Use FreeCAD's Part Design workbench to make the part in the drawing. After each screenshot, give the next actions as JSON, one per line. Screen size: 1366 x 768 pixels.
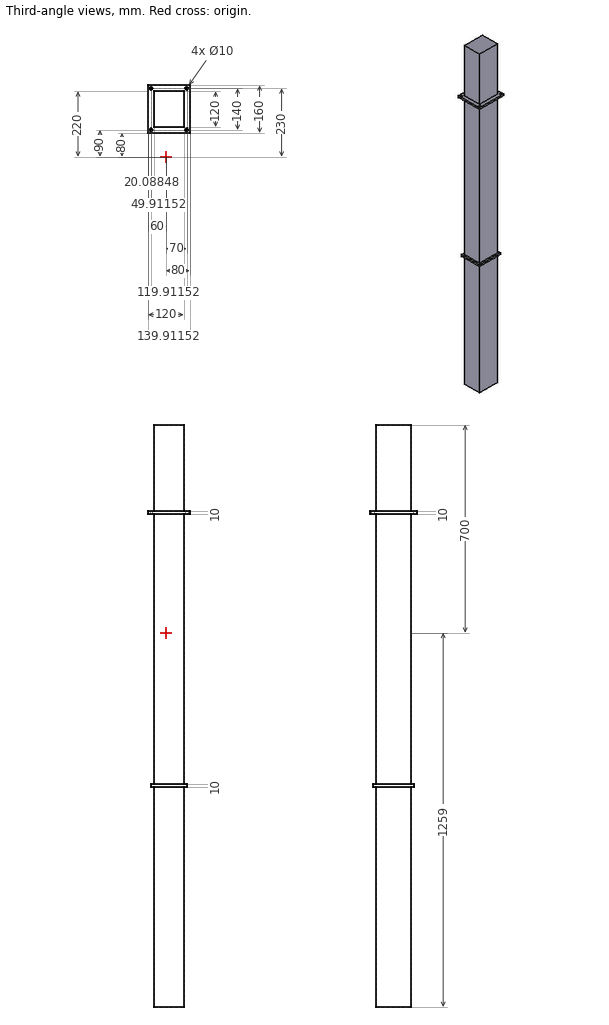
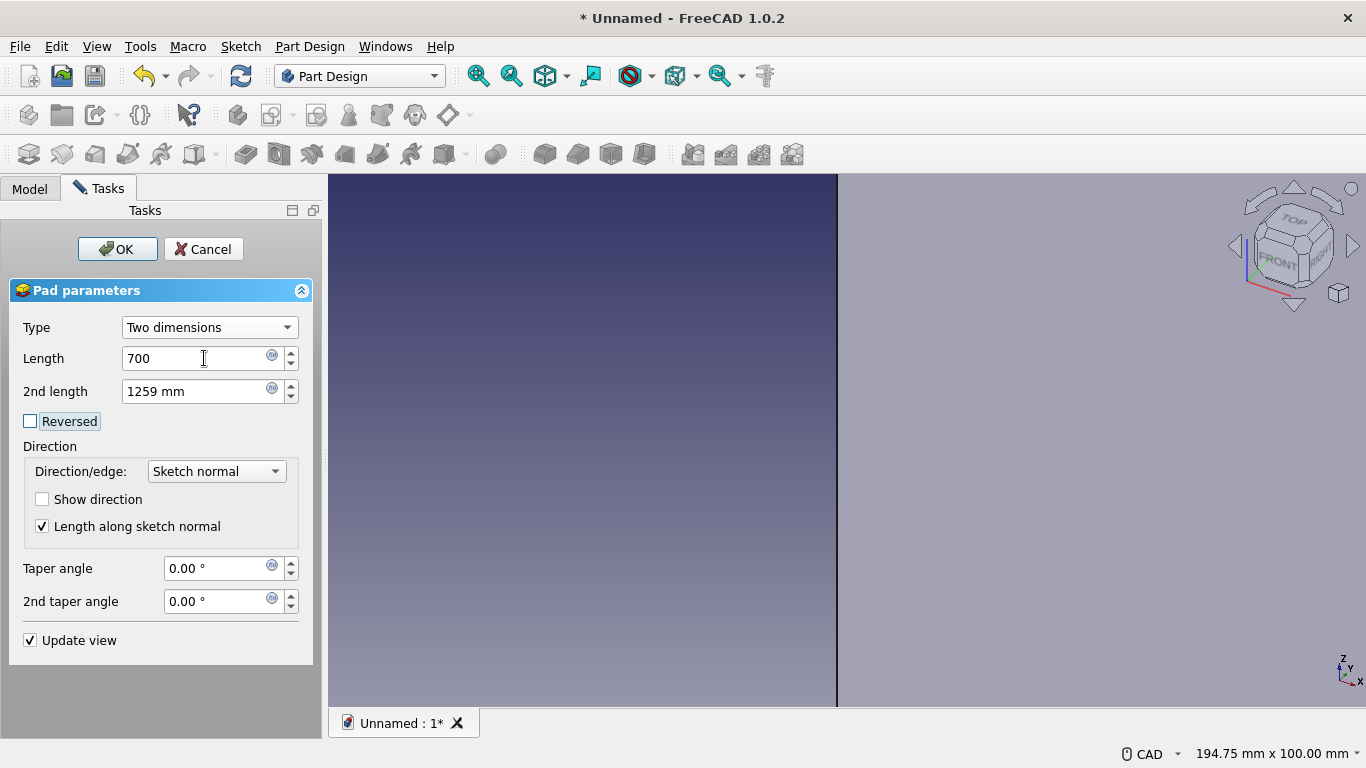
{"action": "left_click", "coordinate": [118, 249]}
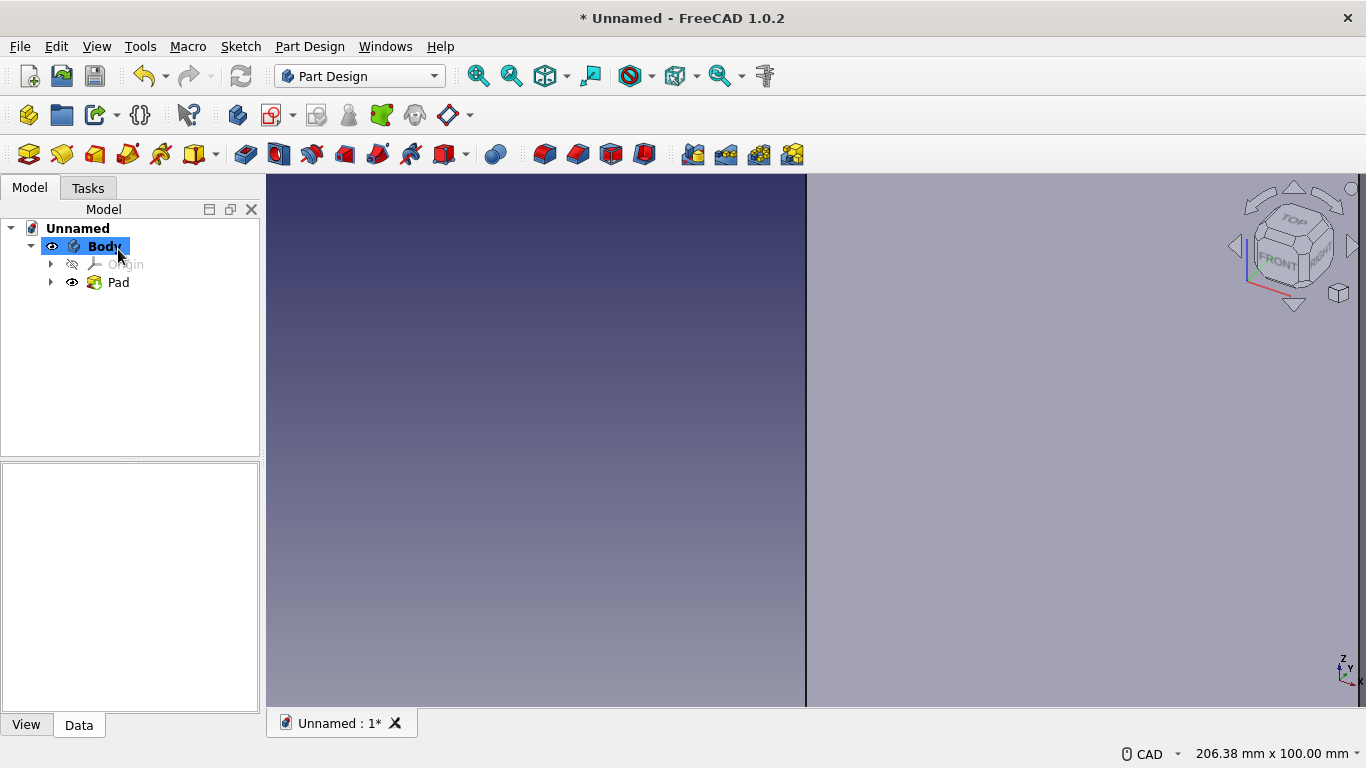
{"action": "key", "text": "v f"}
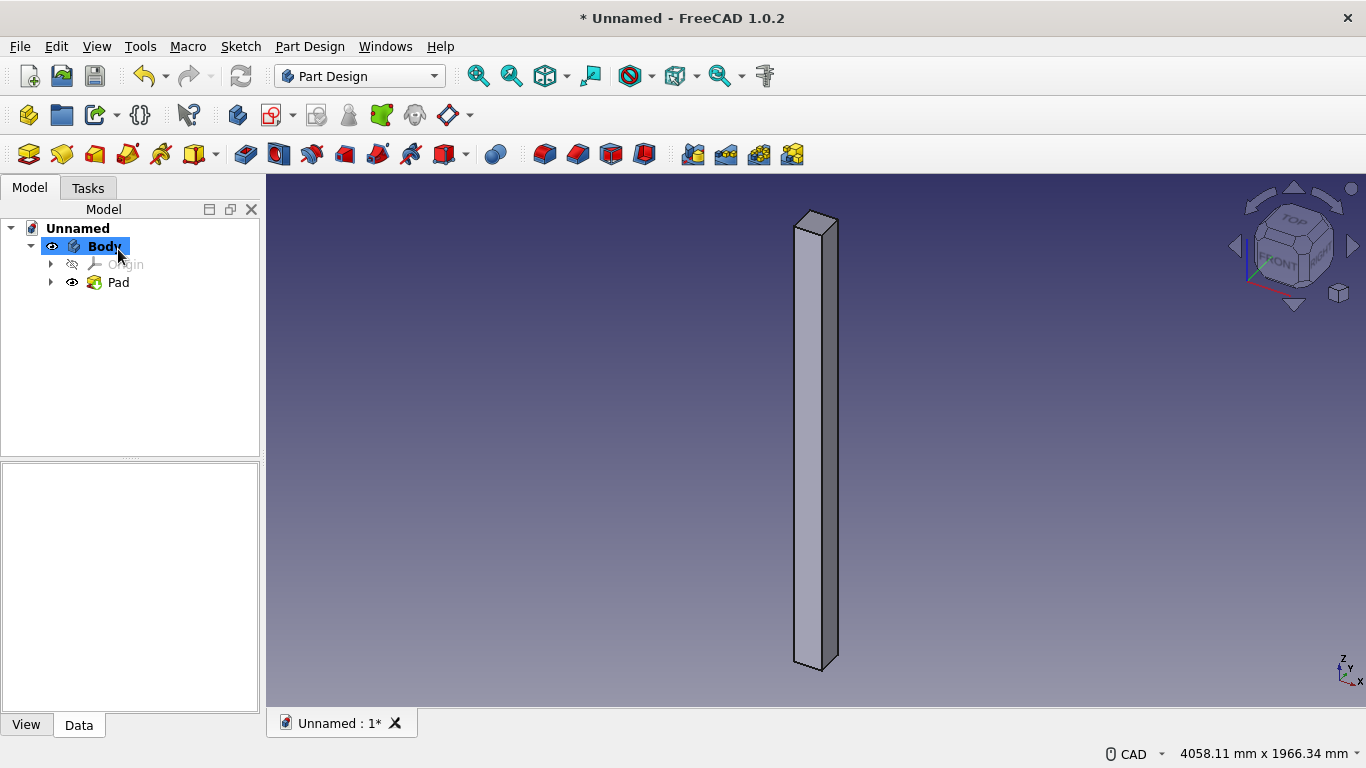
{"action": "left_click", "coordinate": [816, 222]}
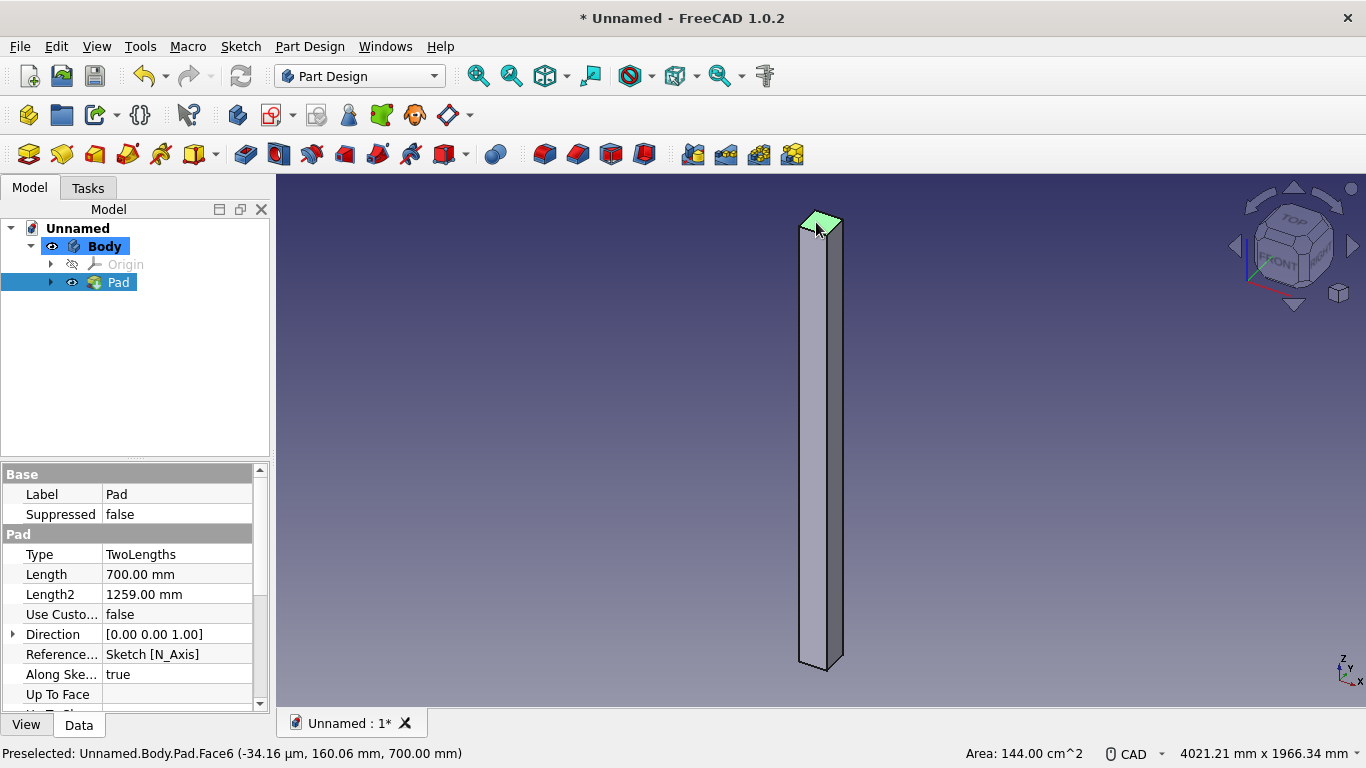
{"action": "left_click", "coordinate": [270, 116]}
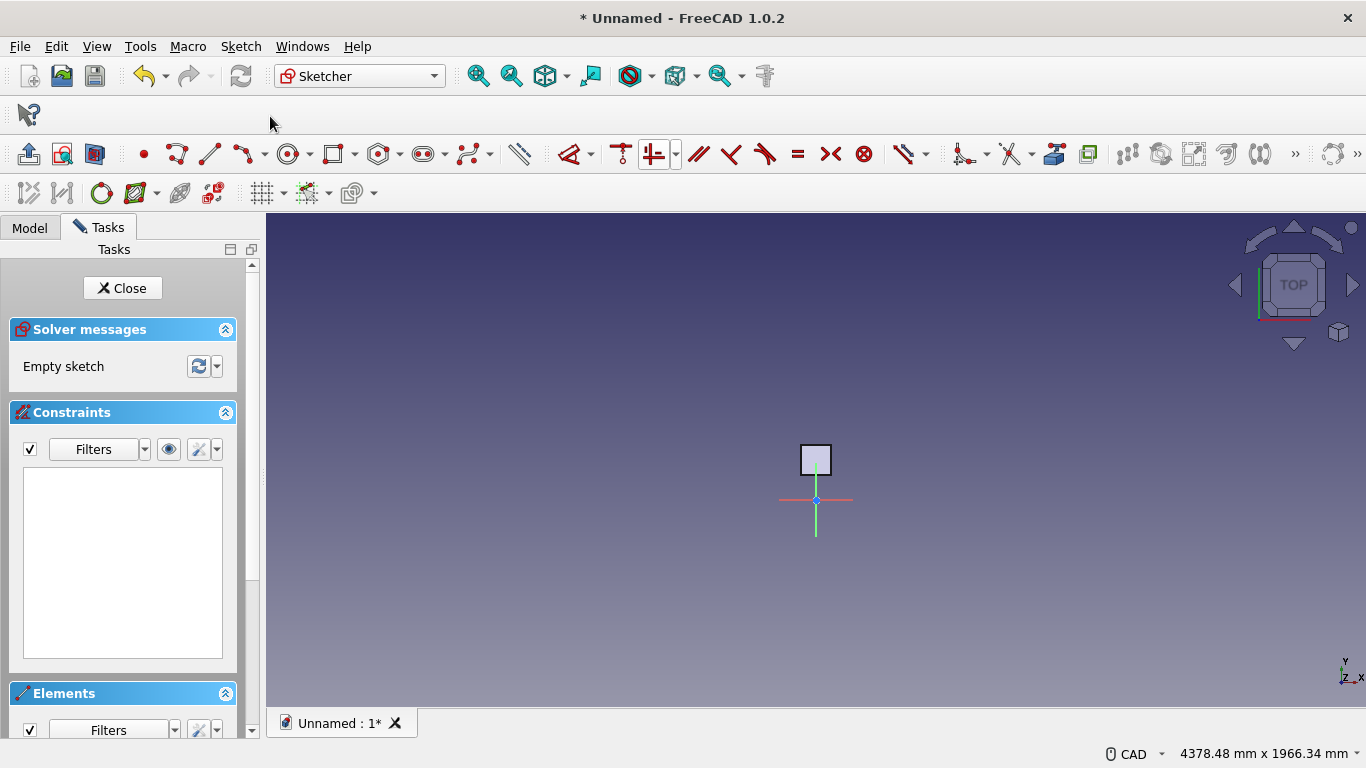
{"action": "scroll", "coordinate": [821, 475], "scroll_direction": "up", "scroll_amount": 9}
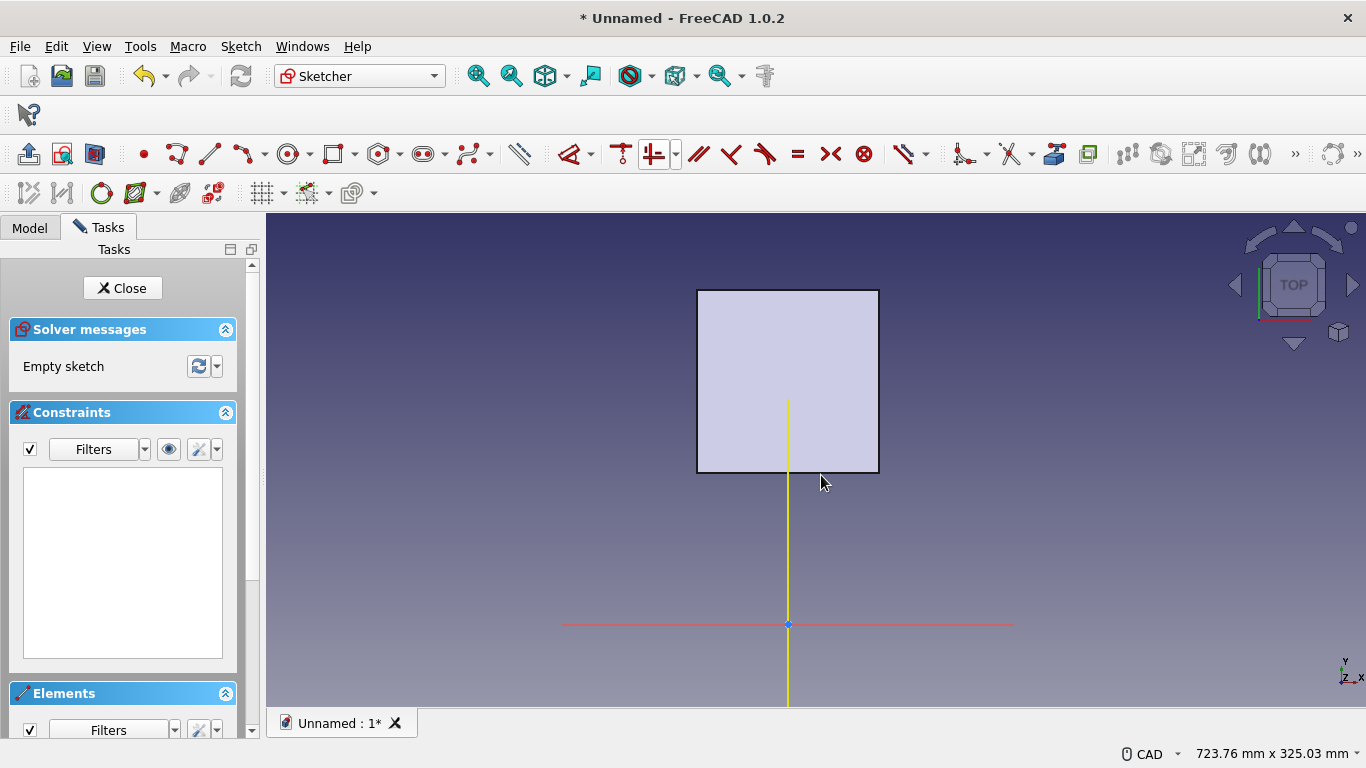
{"action": "key", "text": "g r"}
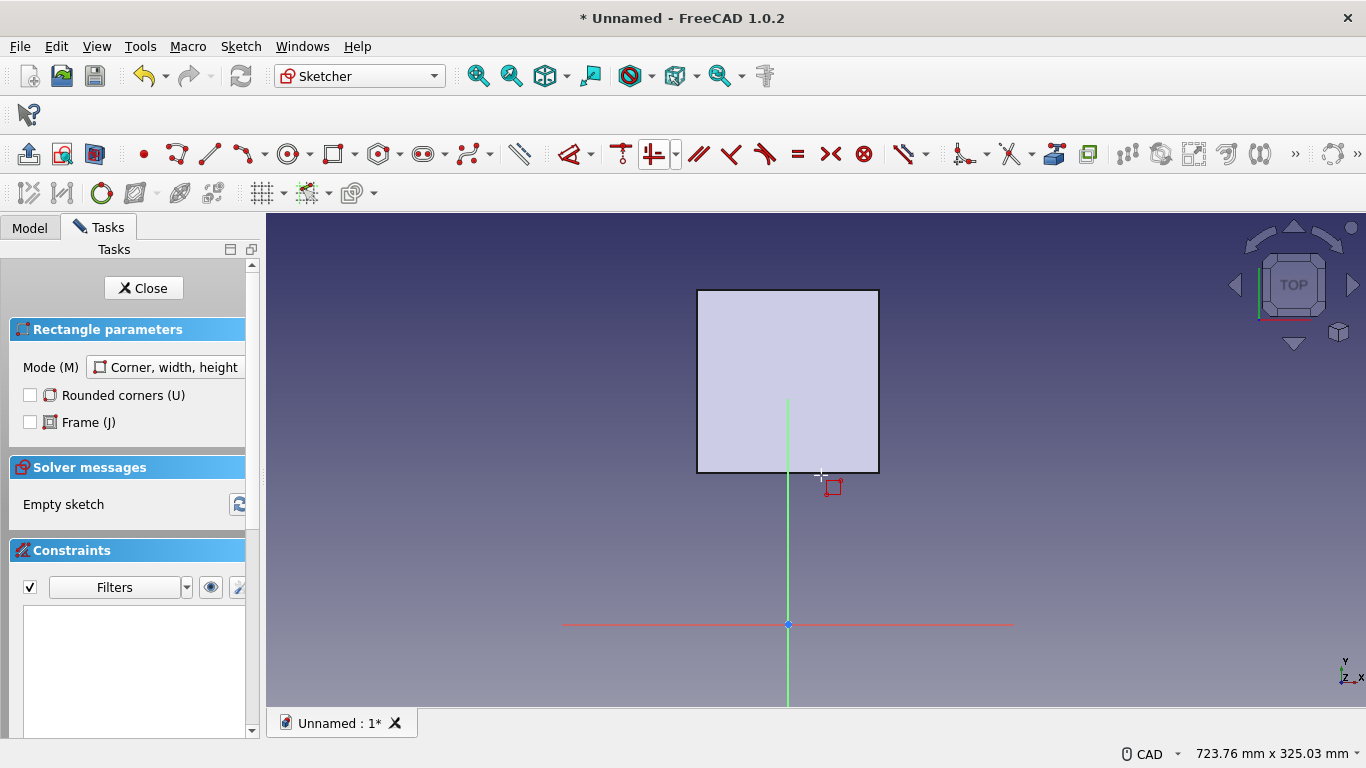
{"action": "left_click", "coordinate": [697, 290]}
{"action": "mouse_move", "coordinate": [728, 473]}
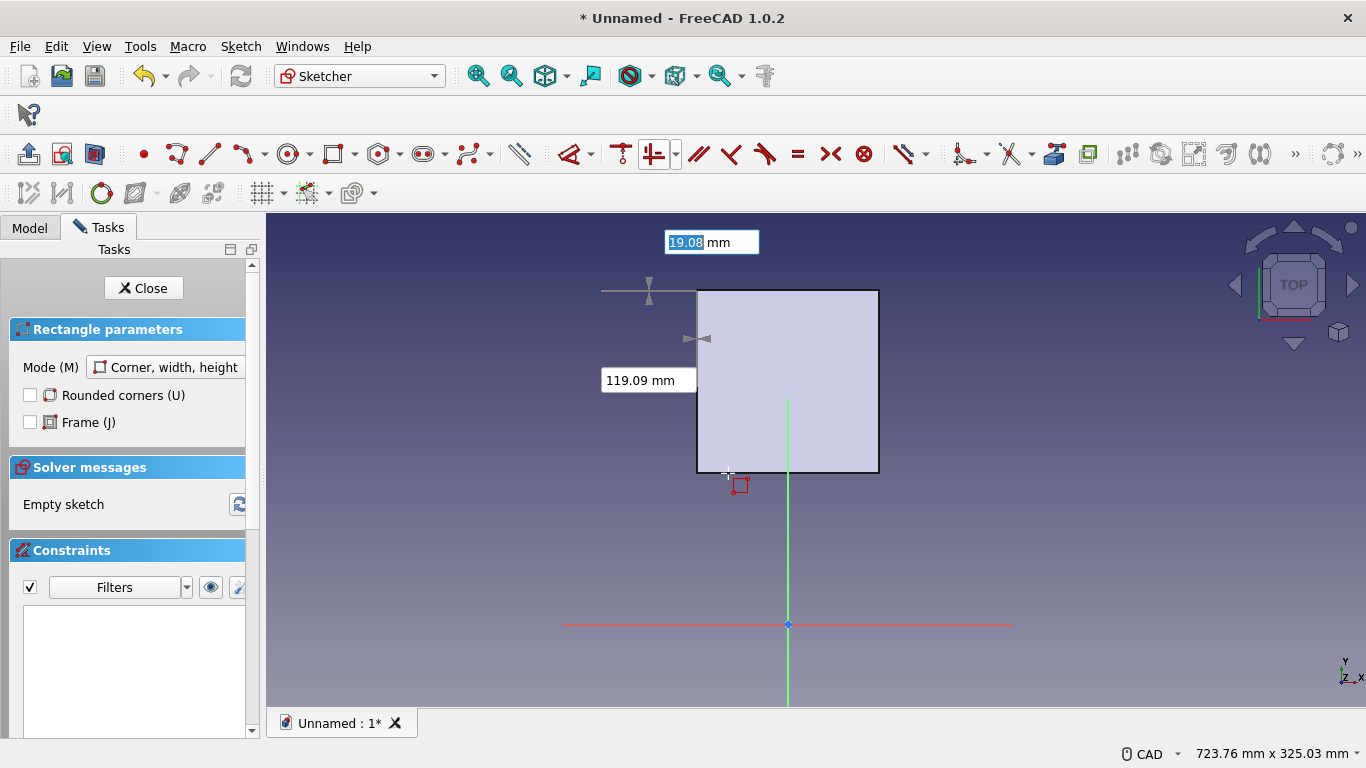
{"action": "type", "text": "20.08848"}
{"action": "key", "text": "Tab"}
{"action": "type", "text": "120"}
{"action": "key", "text": "Return"}
{"action": "key", "text": "Escape"}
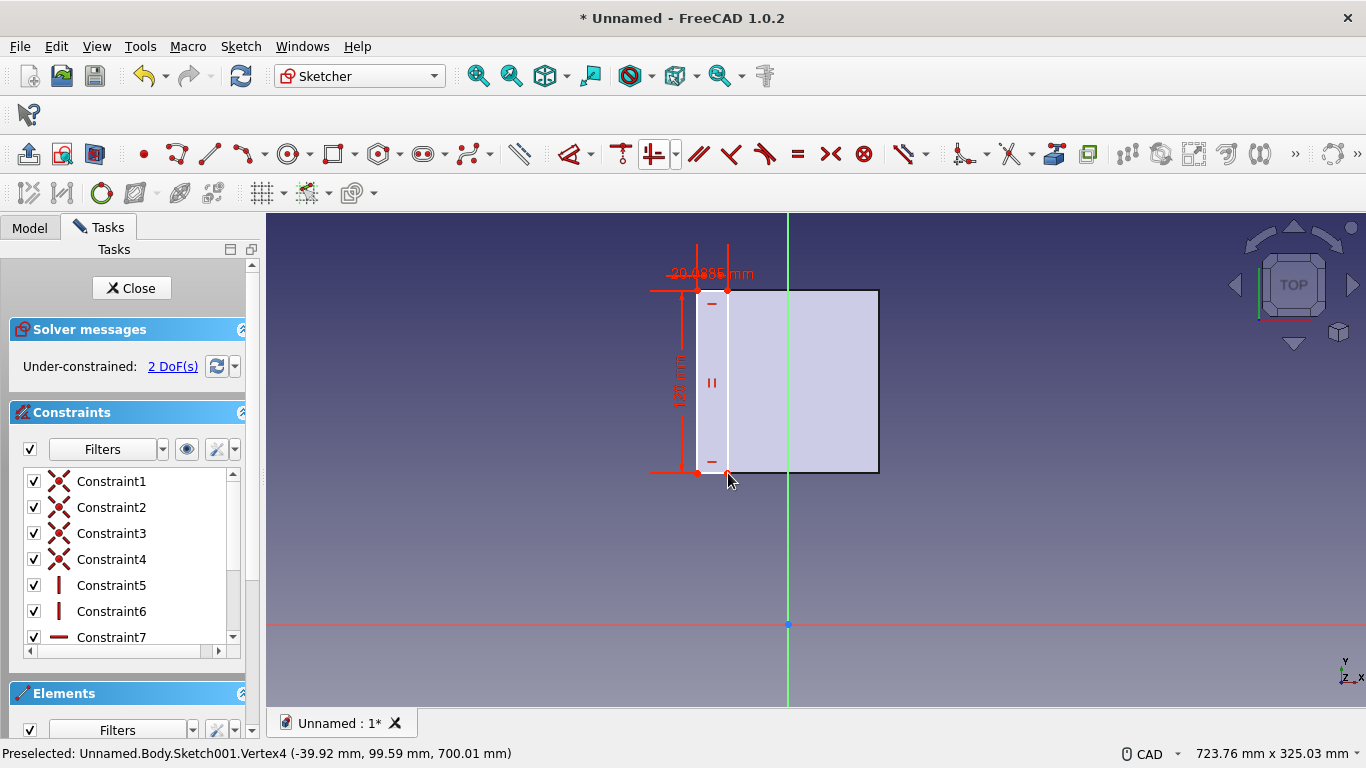
{"action": "left_click", "coordinate": [568, 154]}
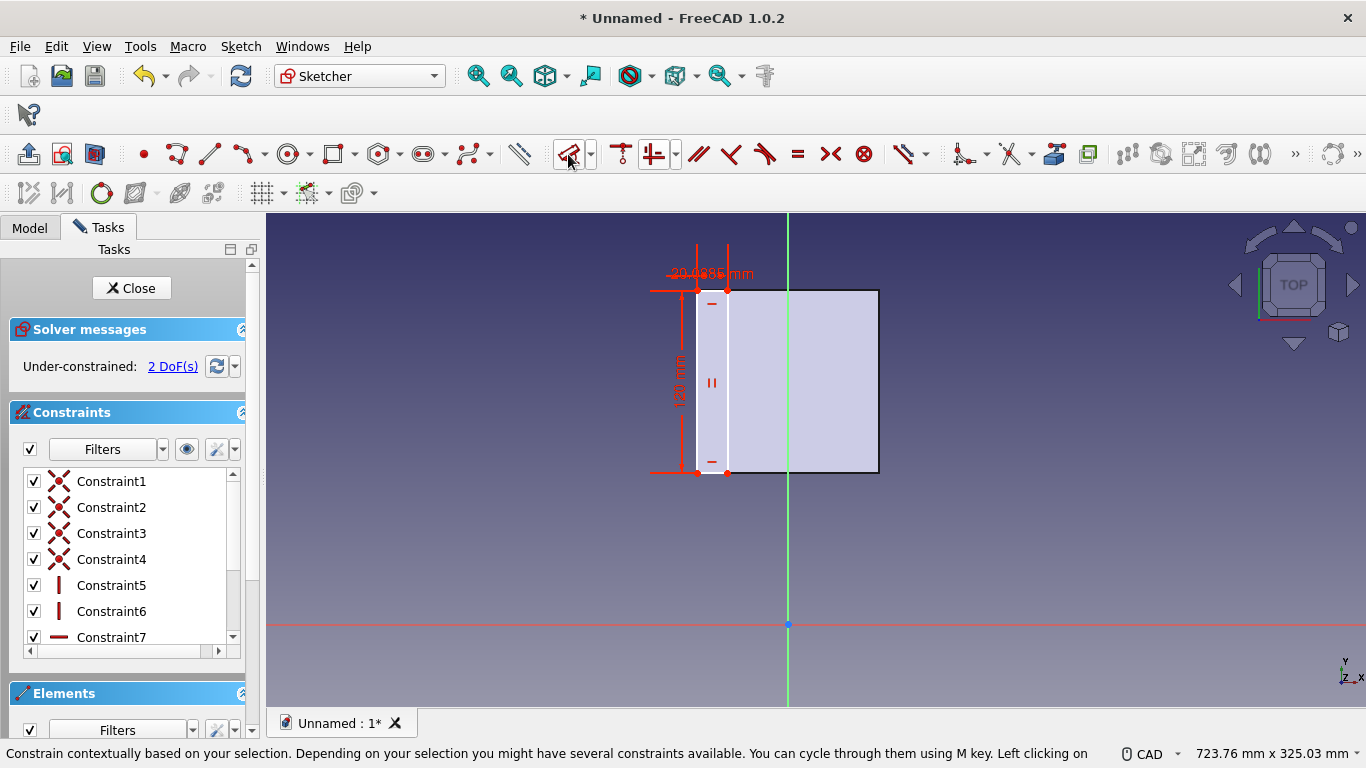
{"action": "left_click", "coordinate": [697, 291]}
{"action": "left_click", "coordinate": [743, 659]}